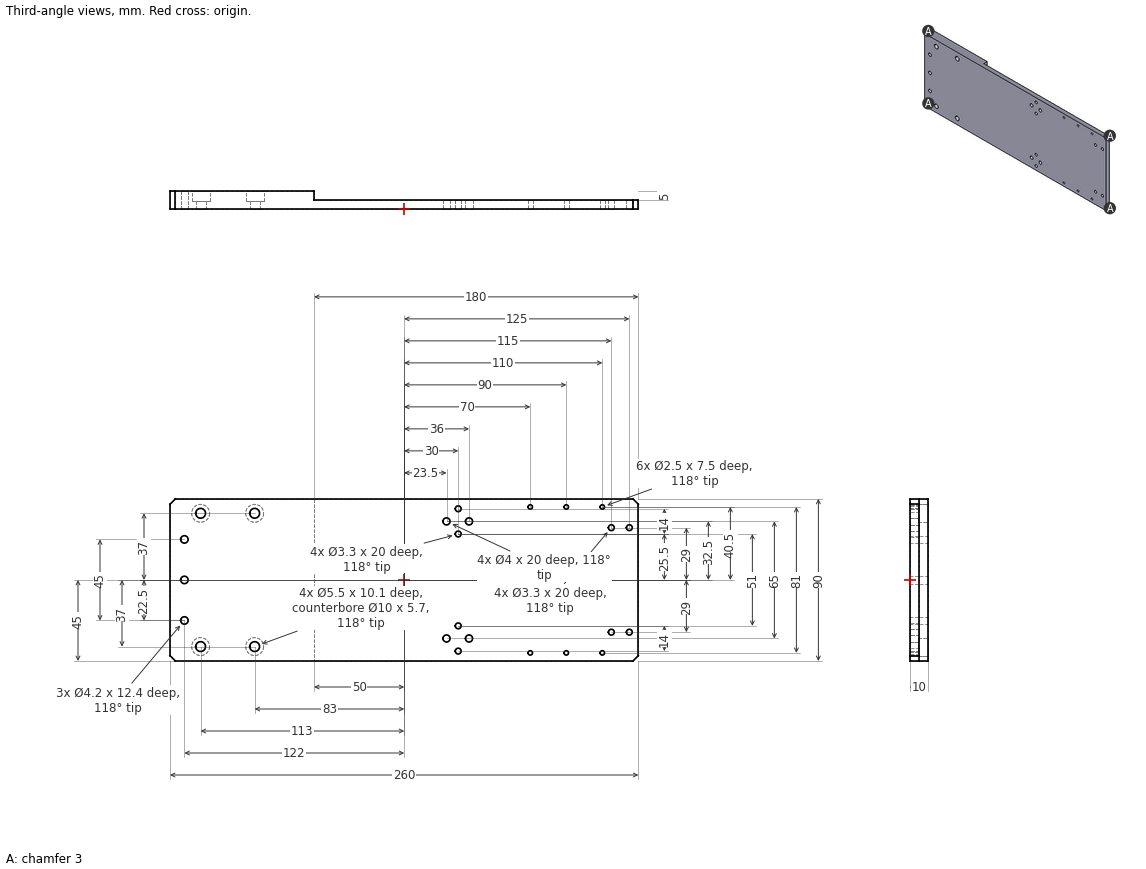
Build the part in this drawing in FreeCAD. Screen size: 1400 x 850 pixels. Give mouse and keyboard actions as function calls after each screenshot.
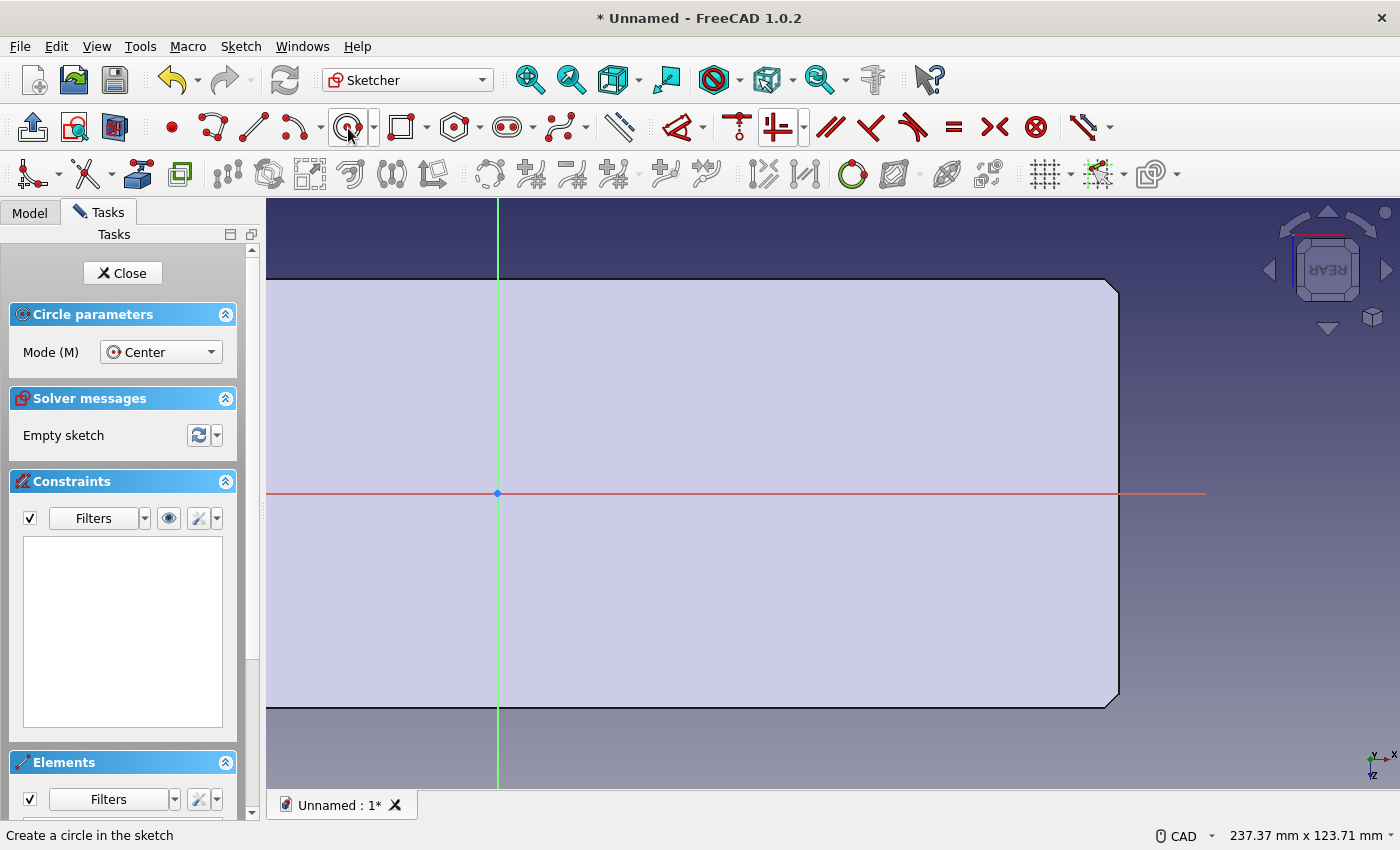
scroll(1023, 687, up, 7)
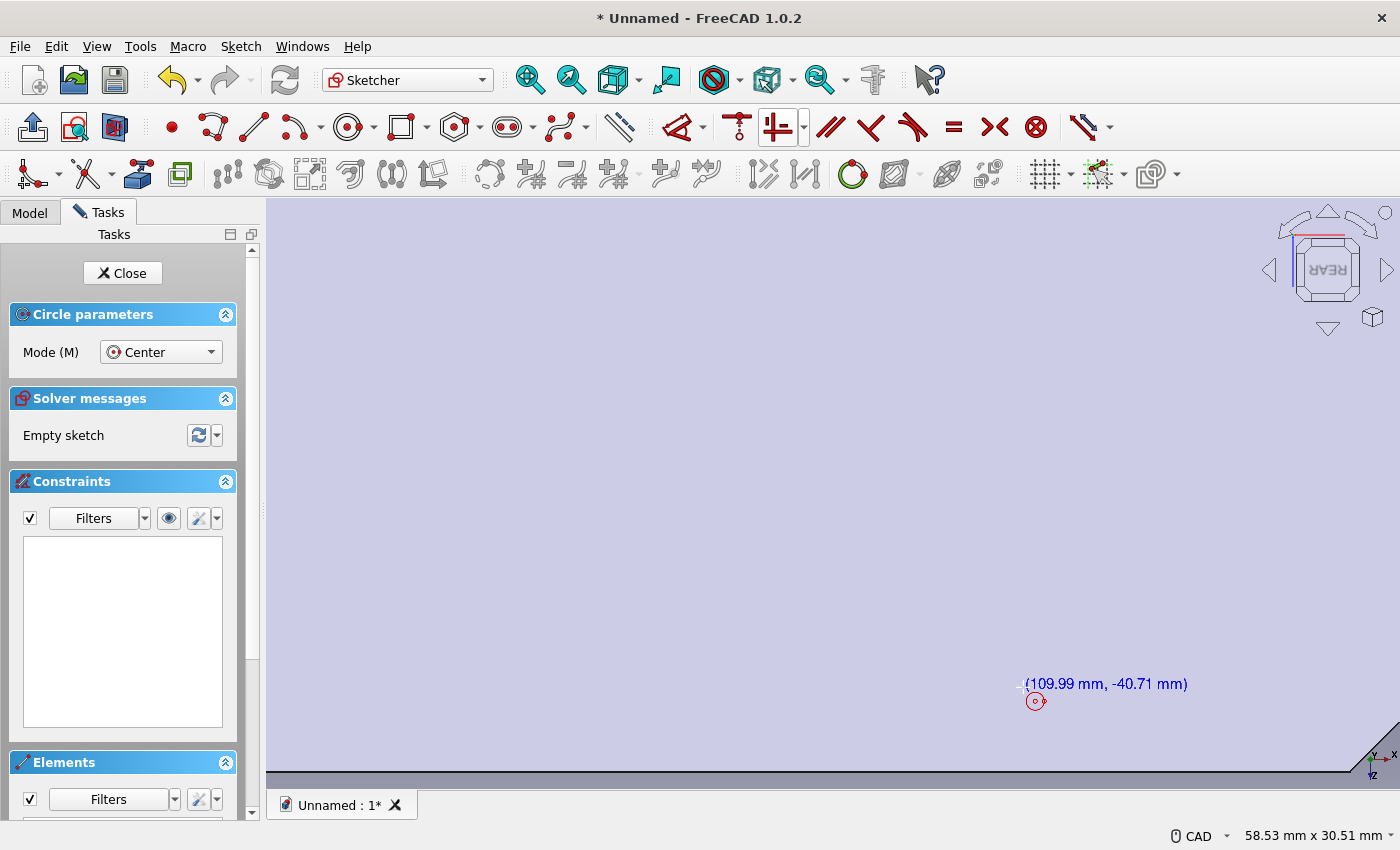
scroll(1025, 688, down, 7)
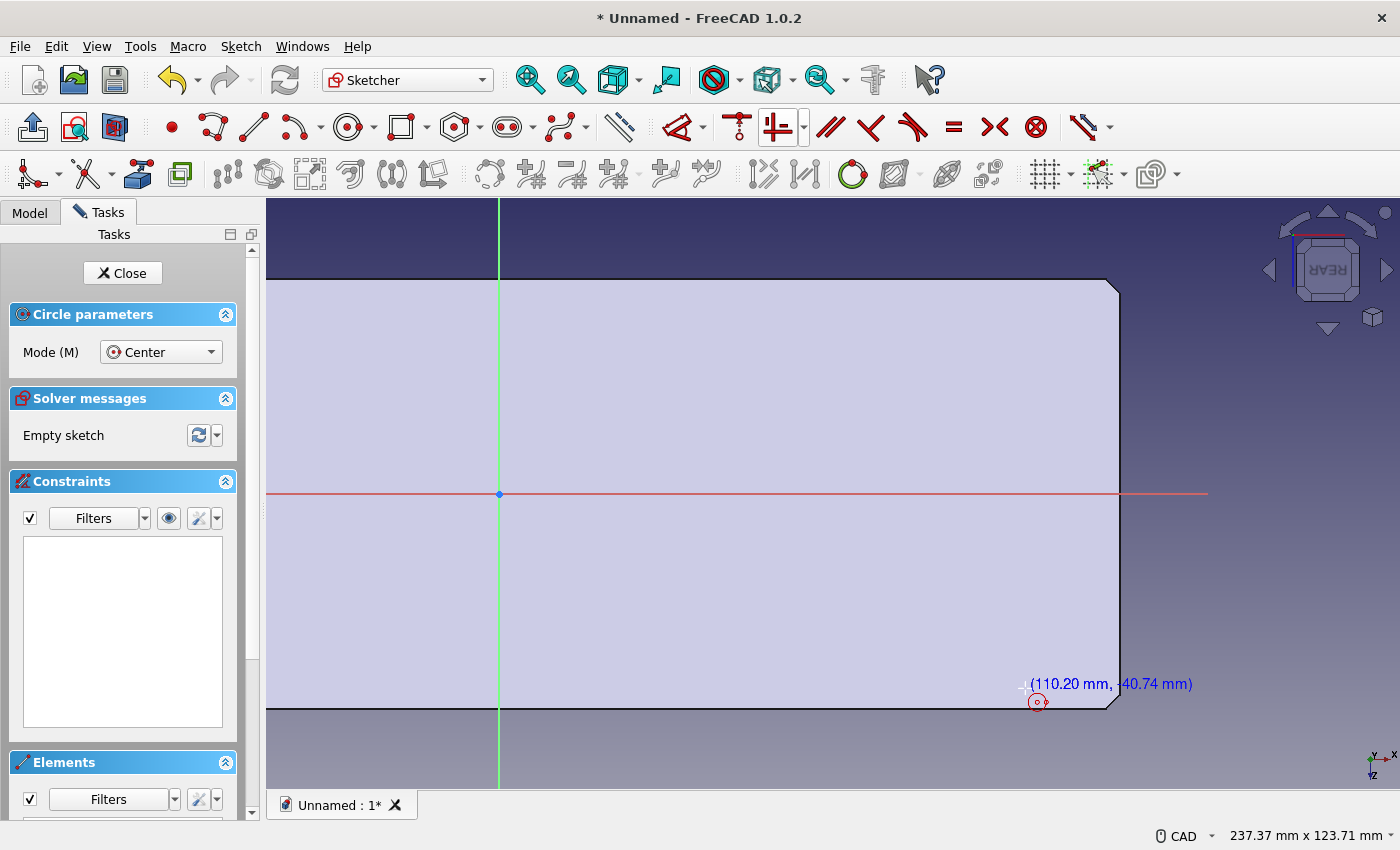
click(1025, 688)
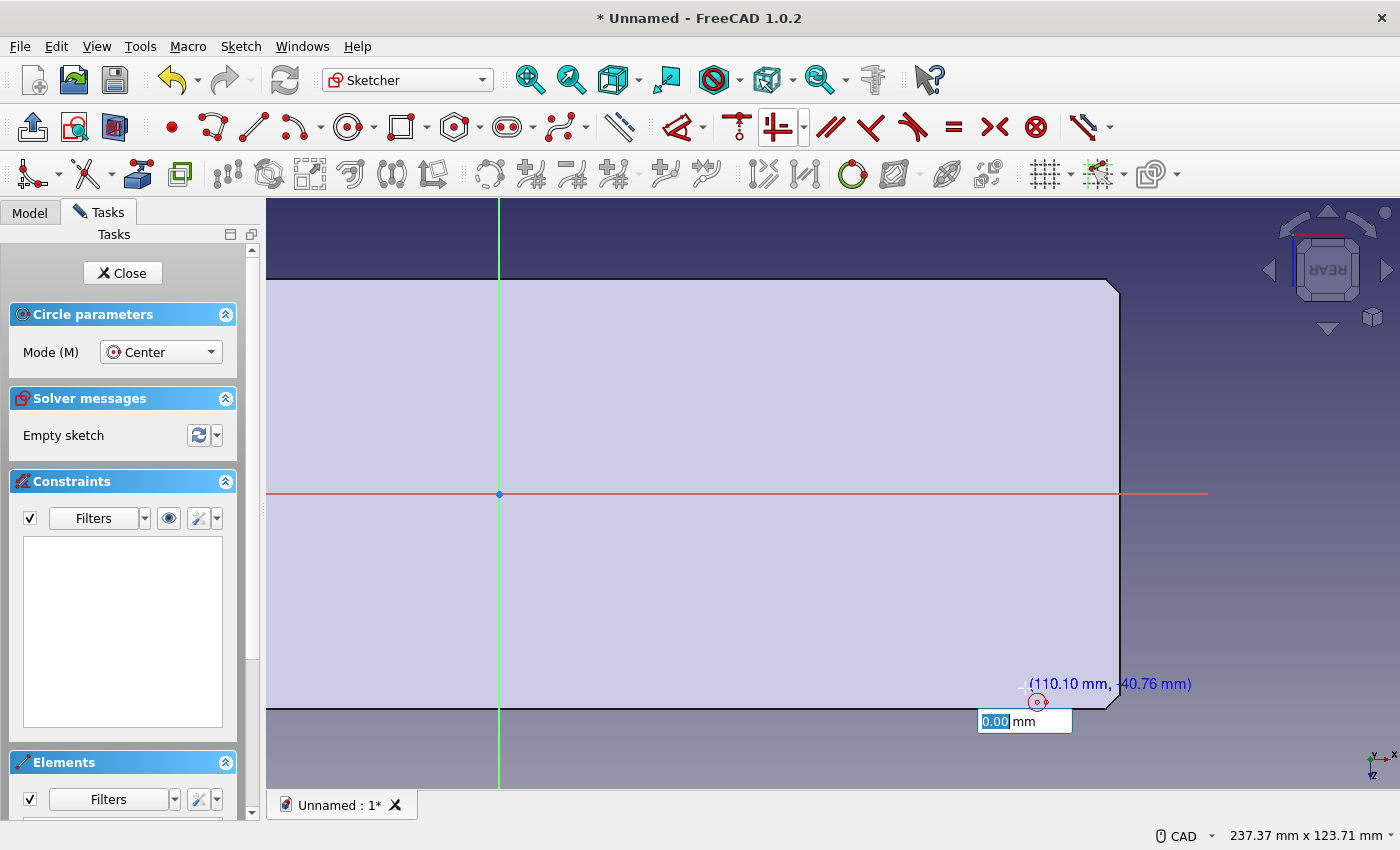
scroll(1029, 684, up, 5)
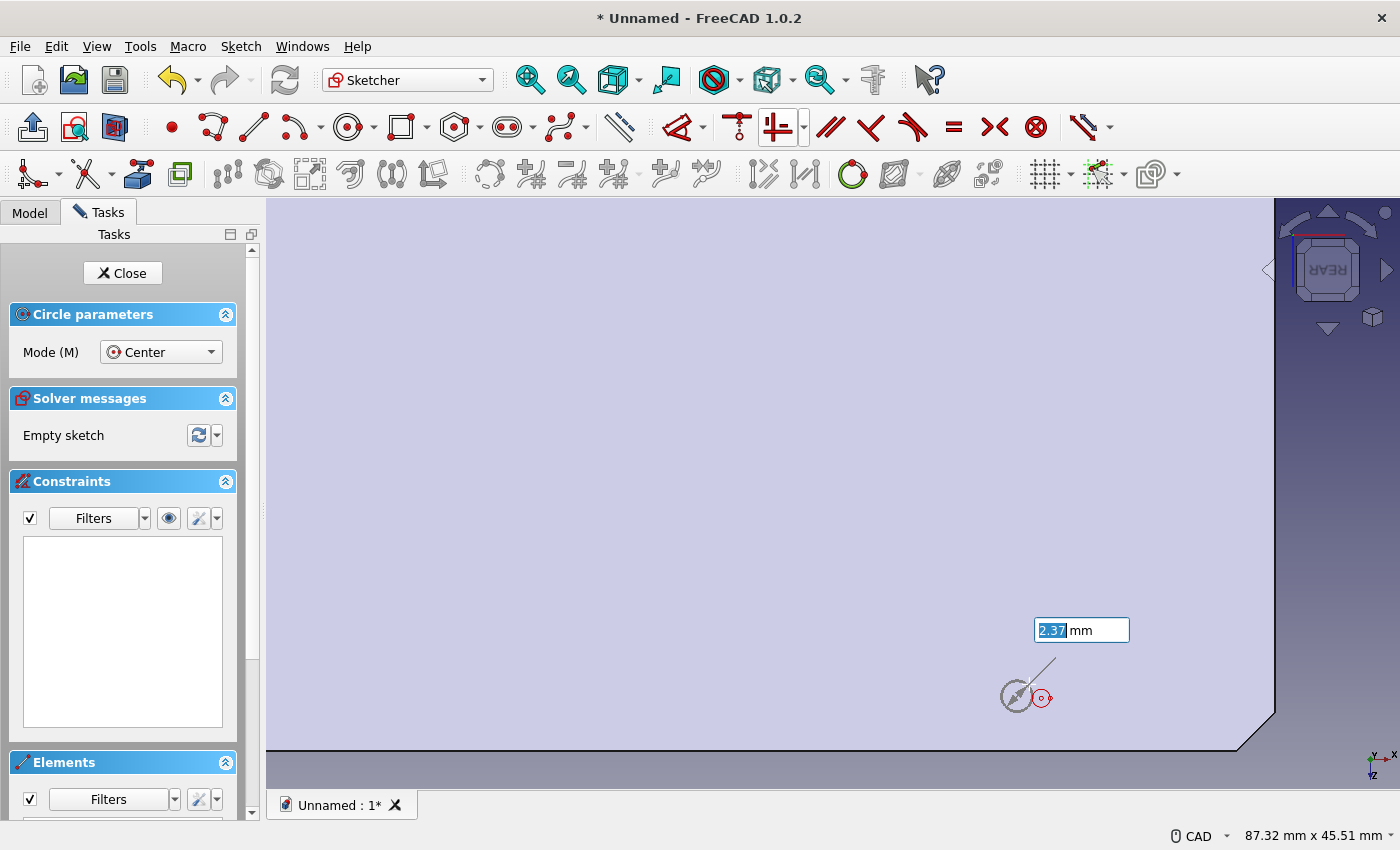
click(1027, 681)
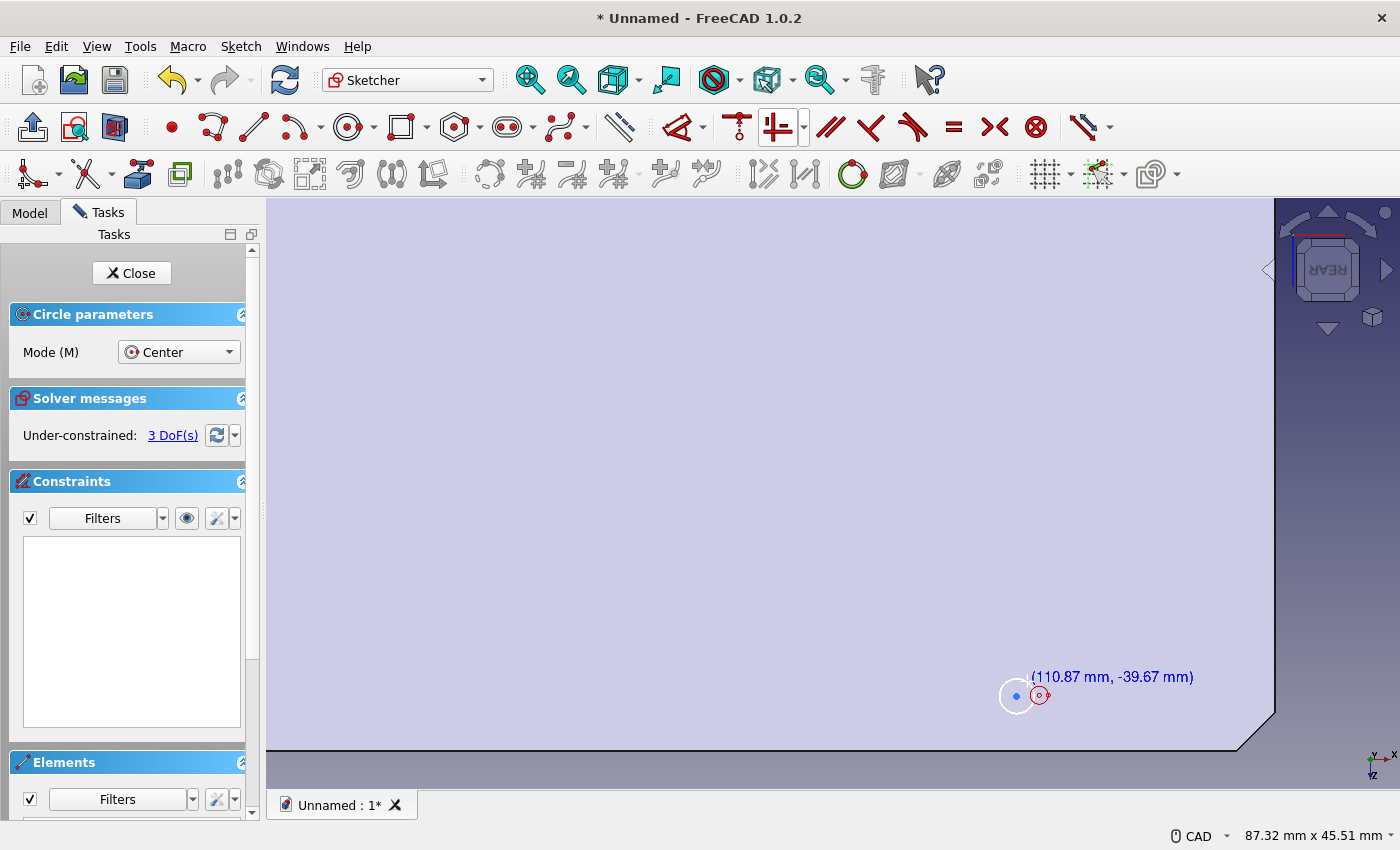
scroll(756, 693, up, 2)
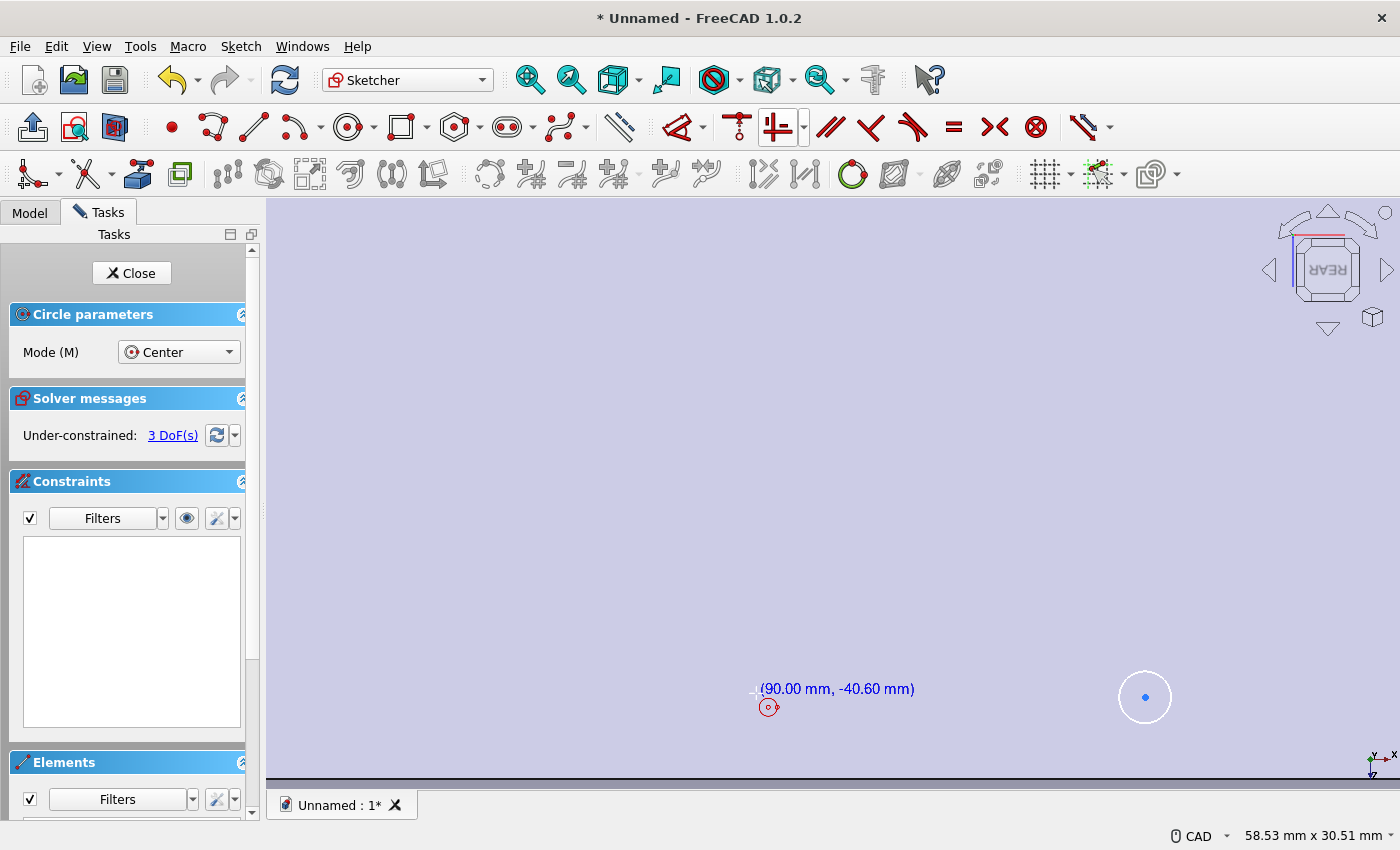
scroll(985, 685, down, 7)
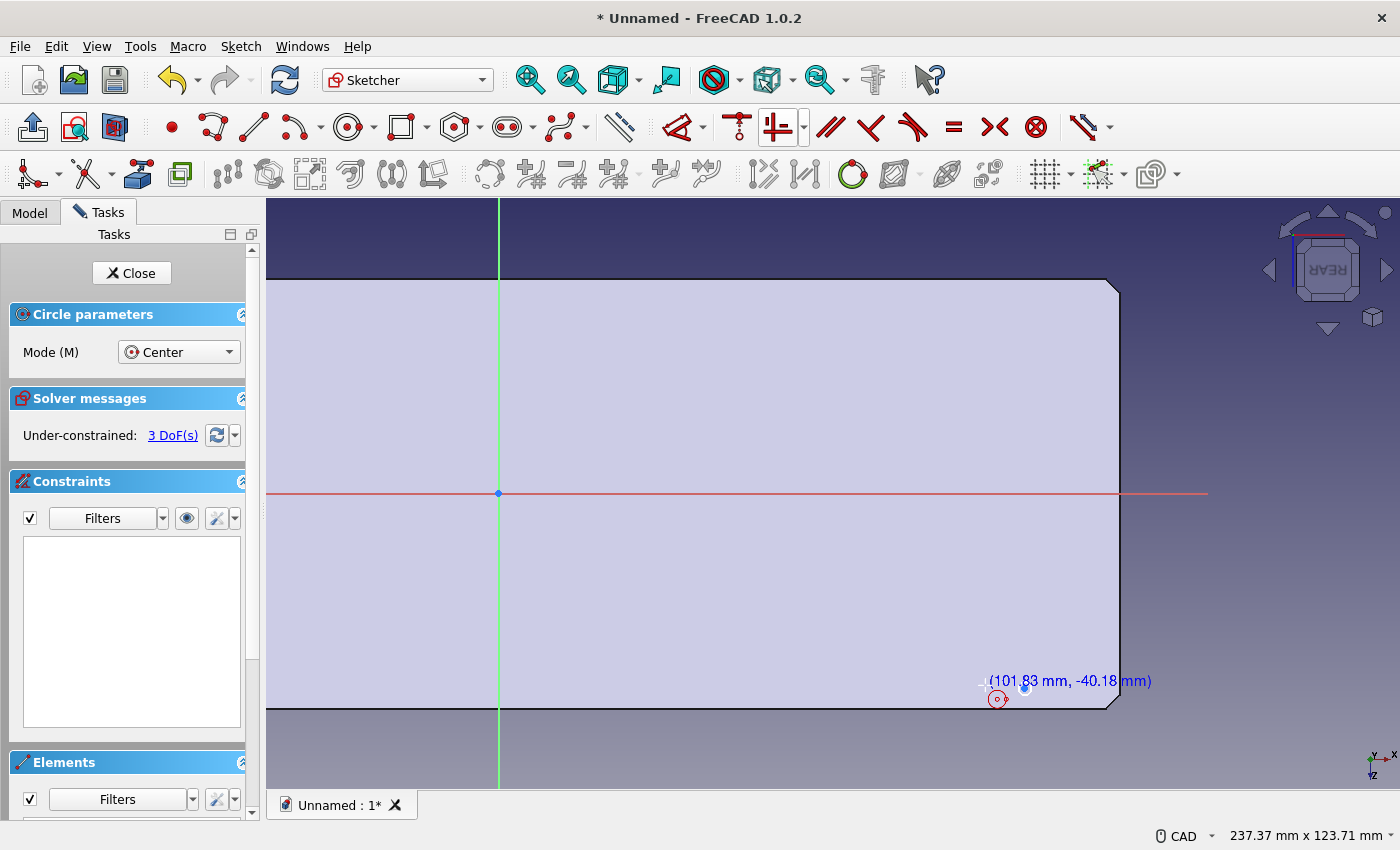
click(929, 687)